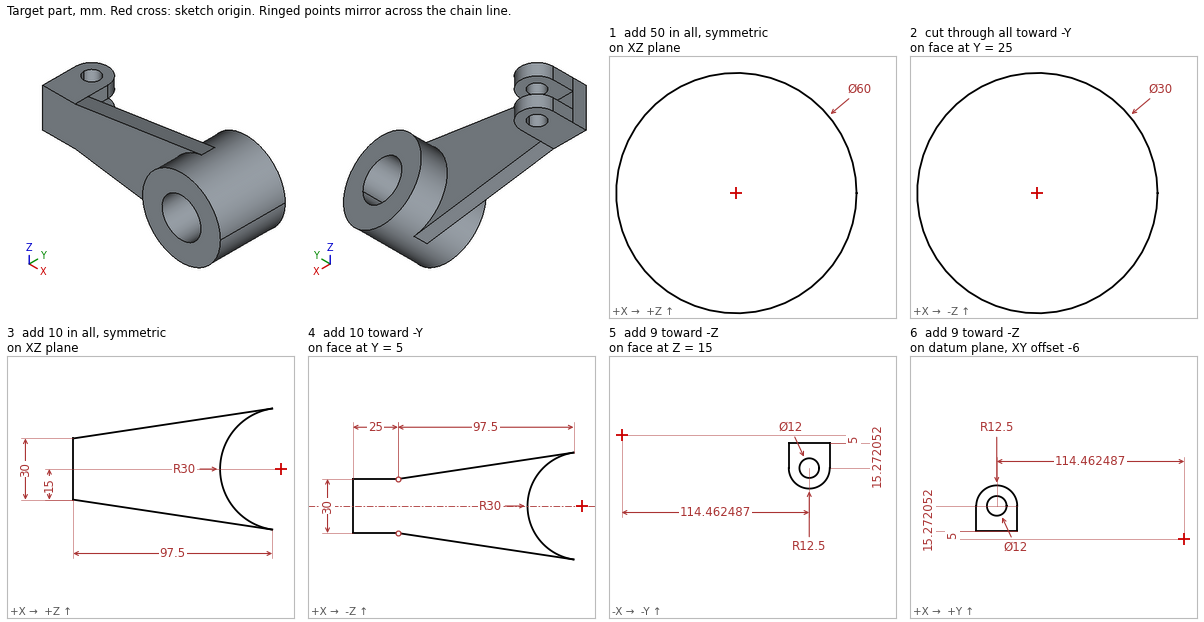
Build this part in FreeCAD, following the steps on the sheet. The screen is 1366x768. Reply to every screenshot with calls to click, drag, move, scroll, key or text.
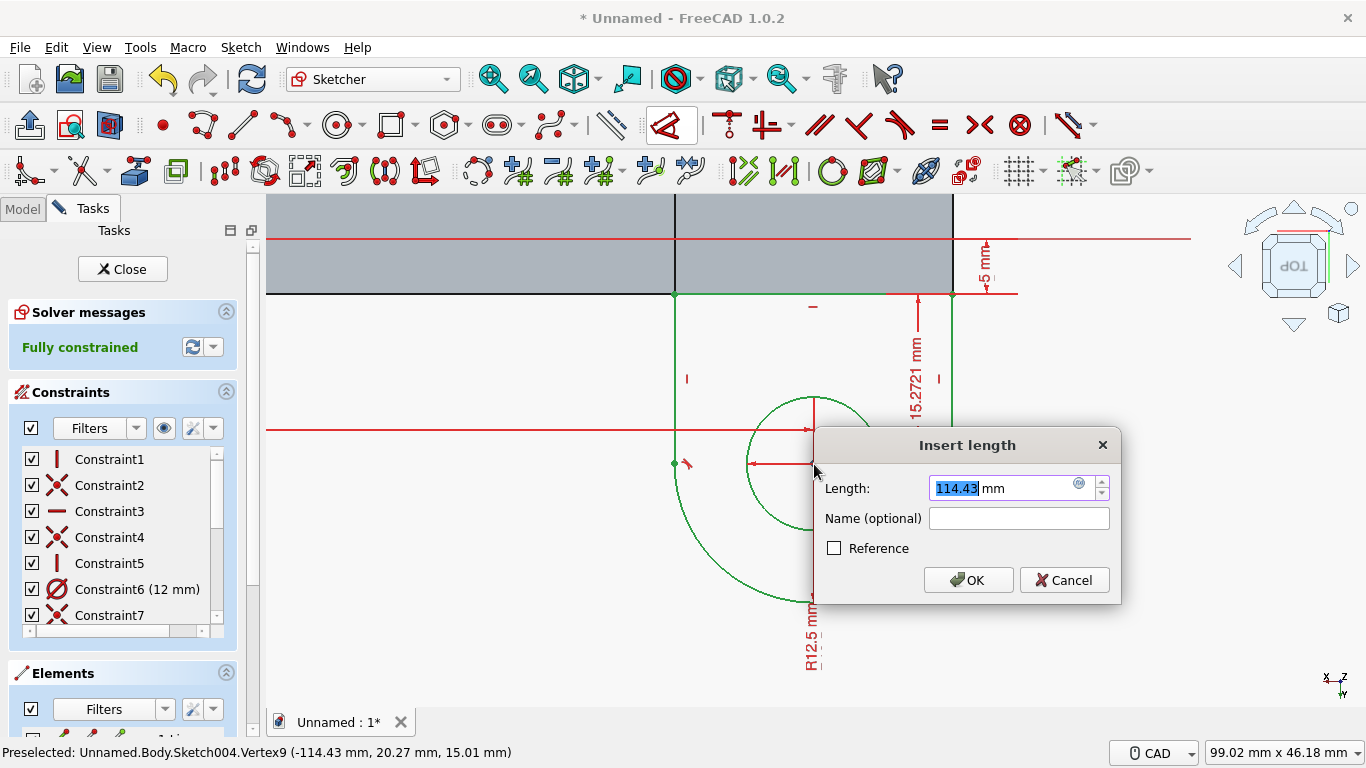
text(114.462487)
key(Return)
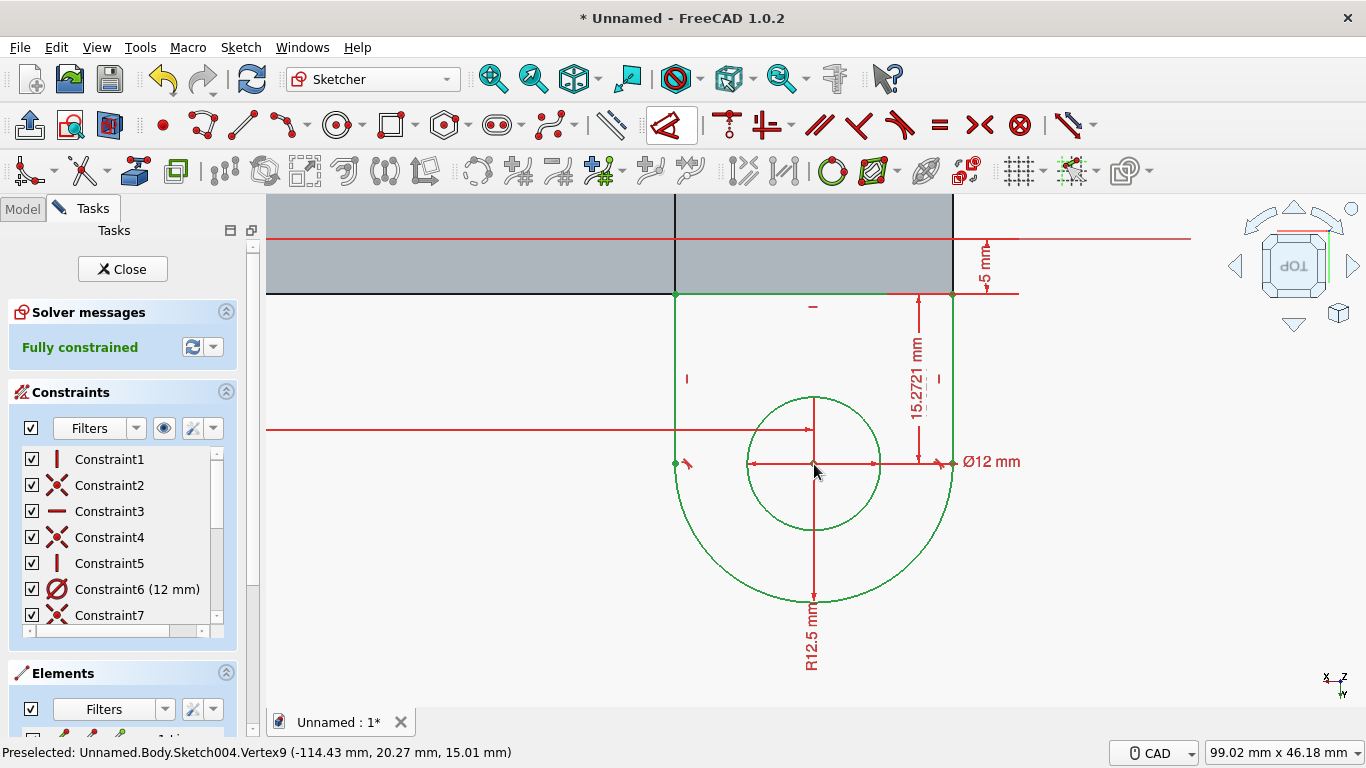
click(123, 269)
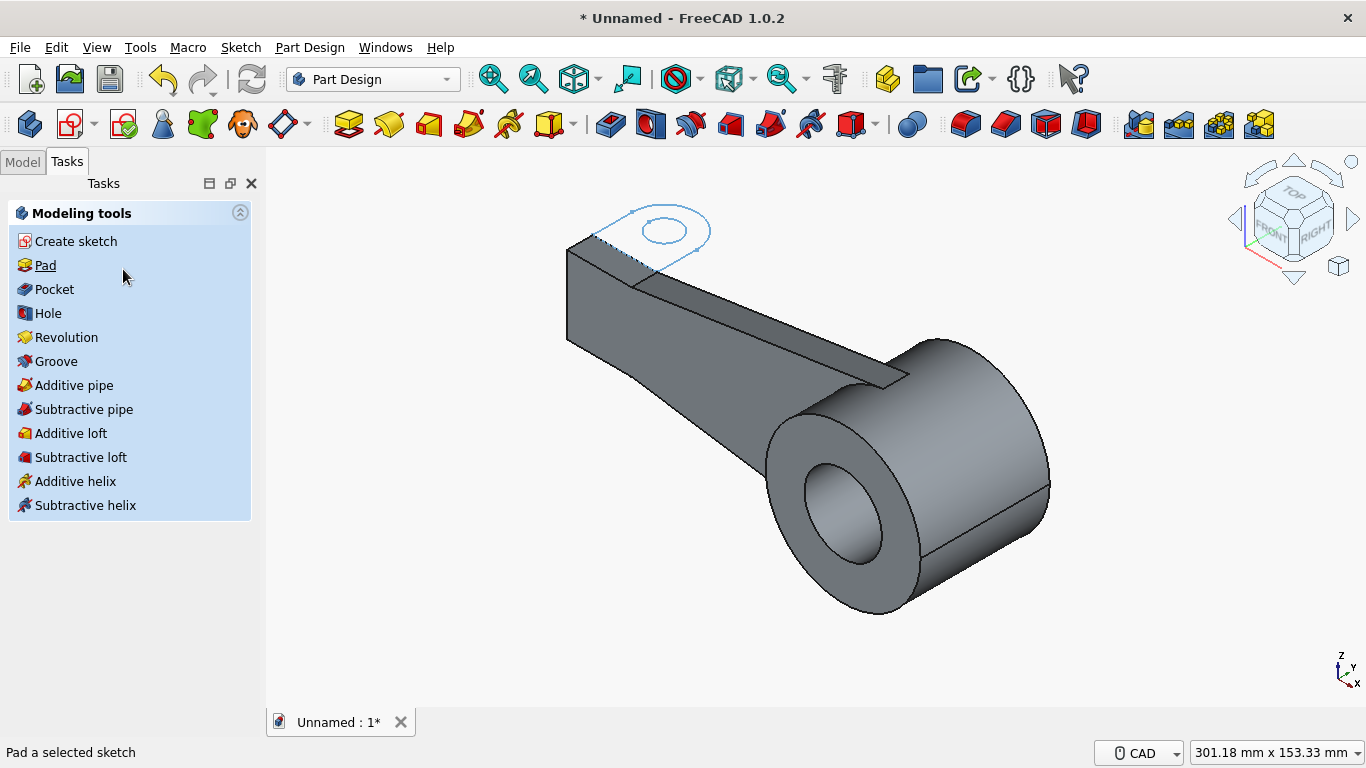
click(350, 124)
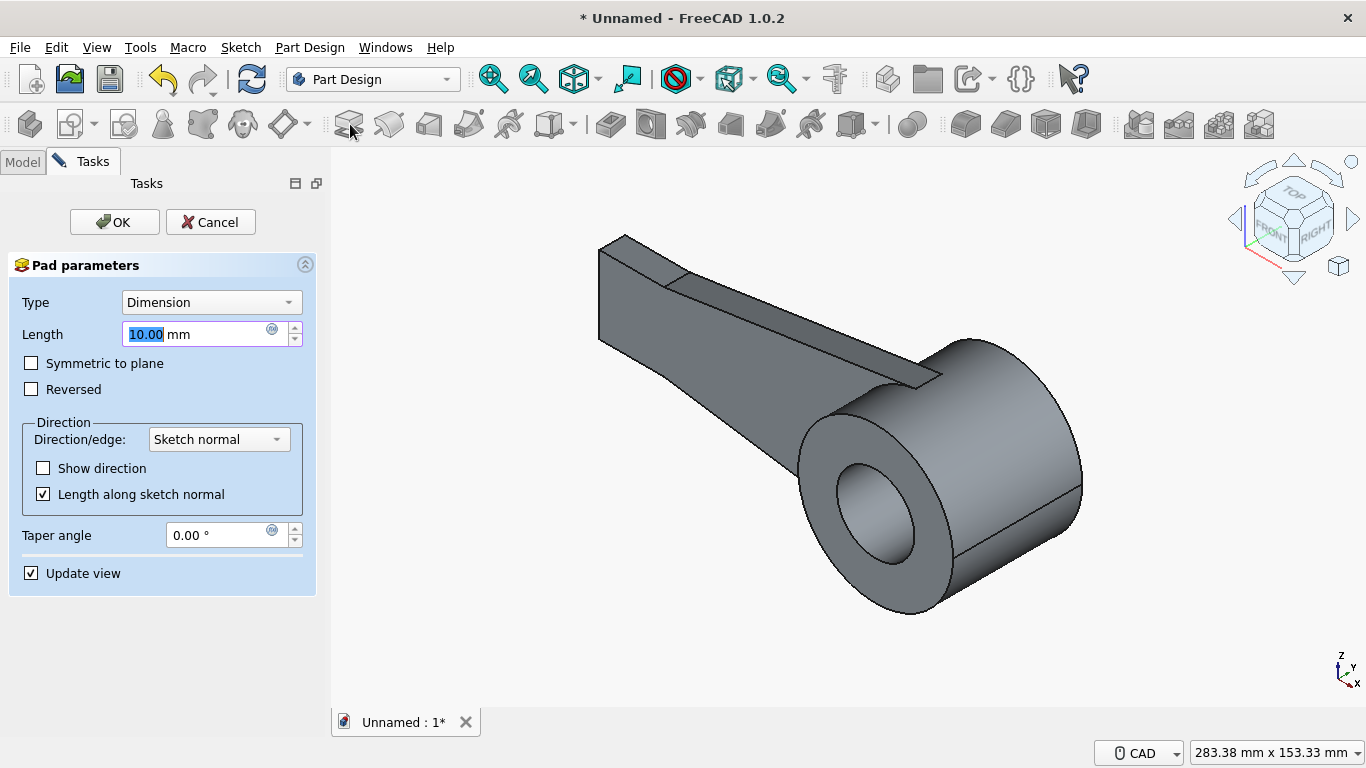
text(9)
key(Tab)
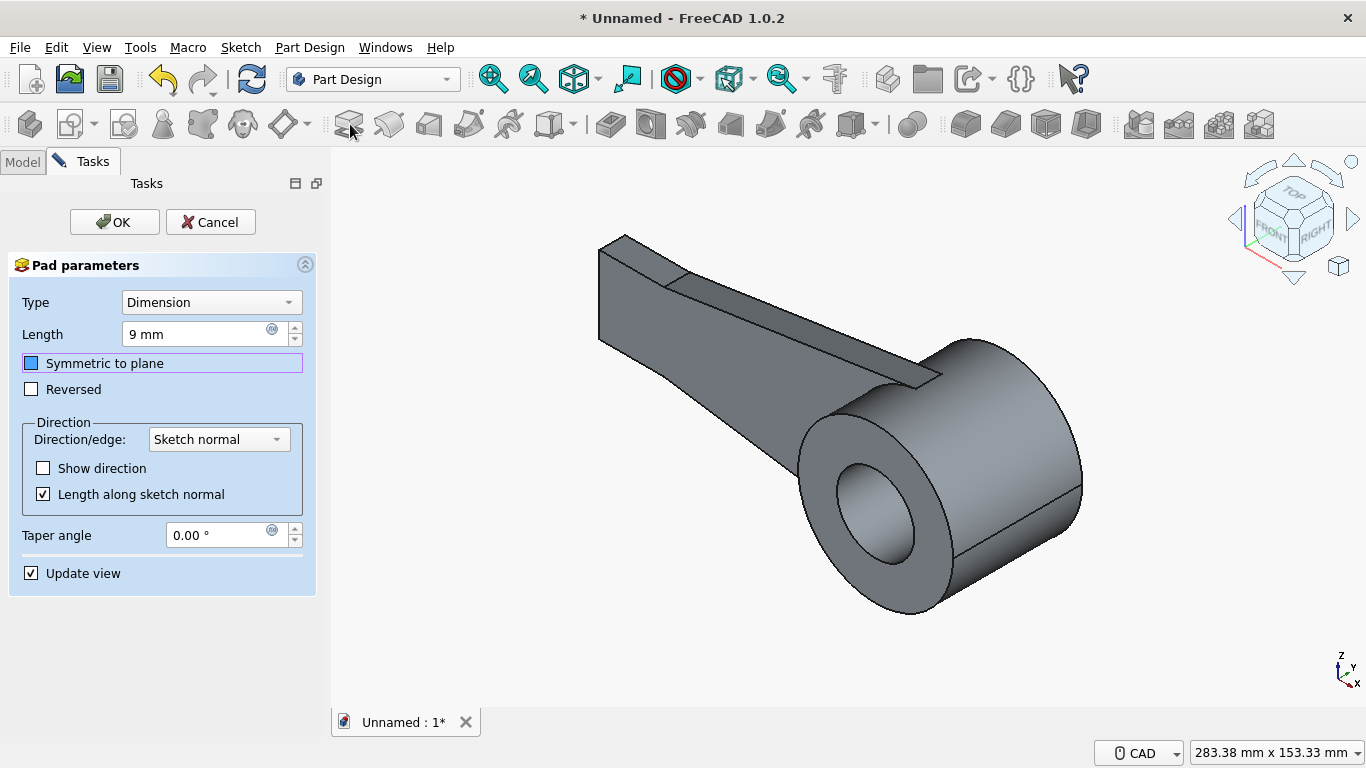
click(30, 389)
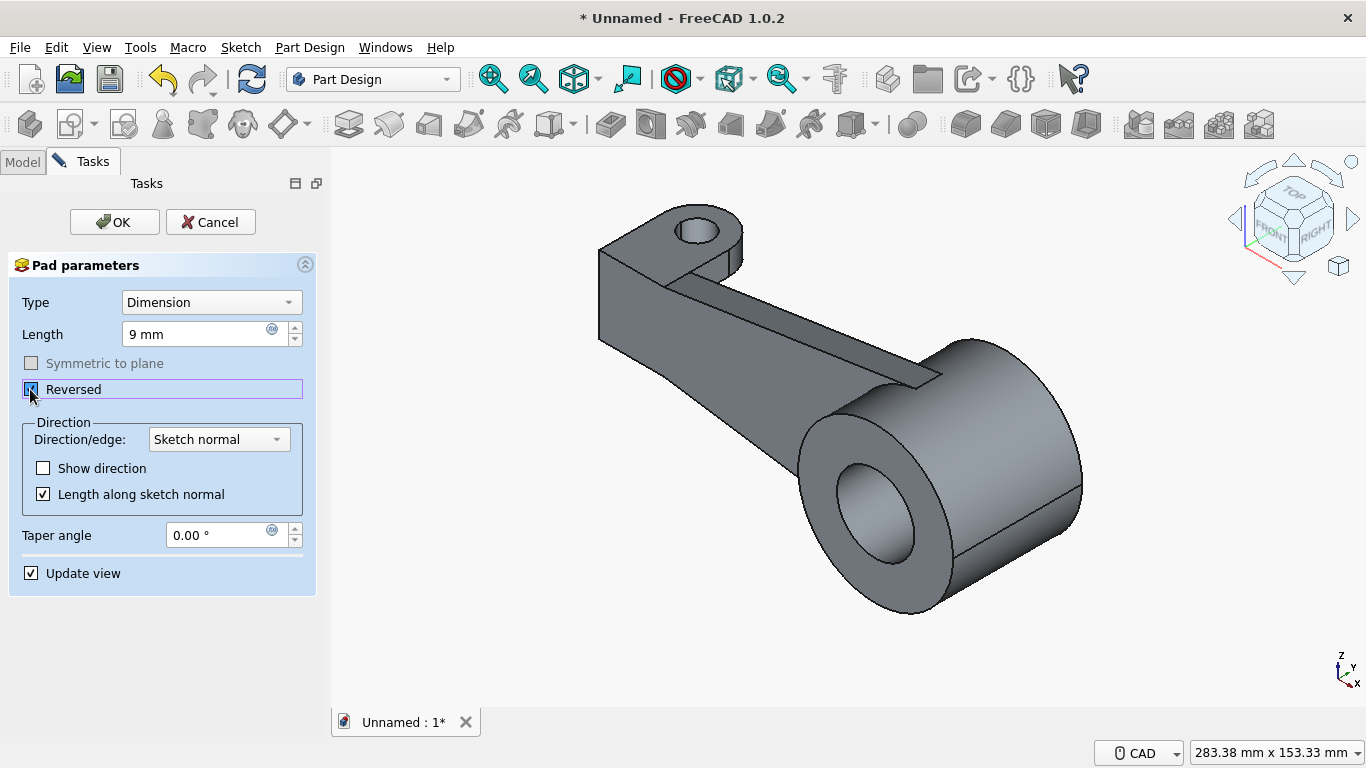
click(115, 222)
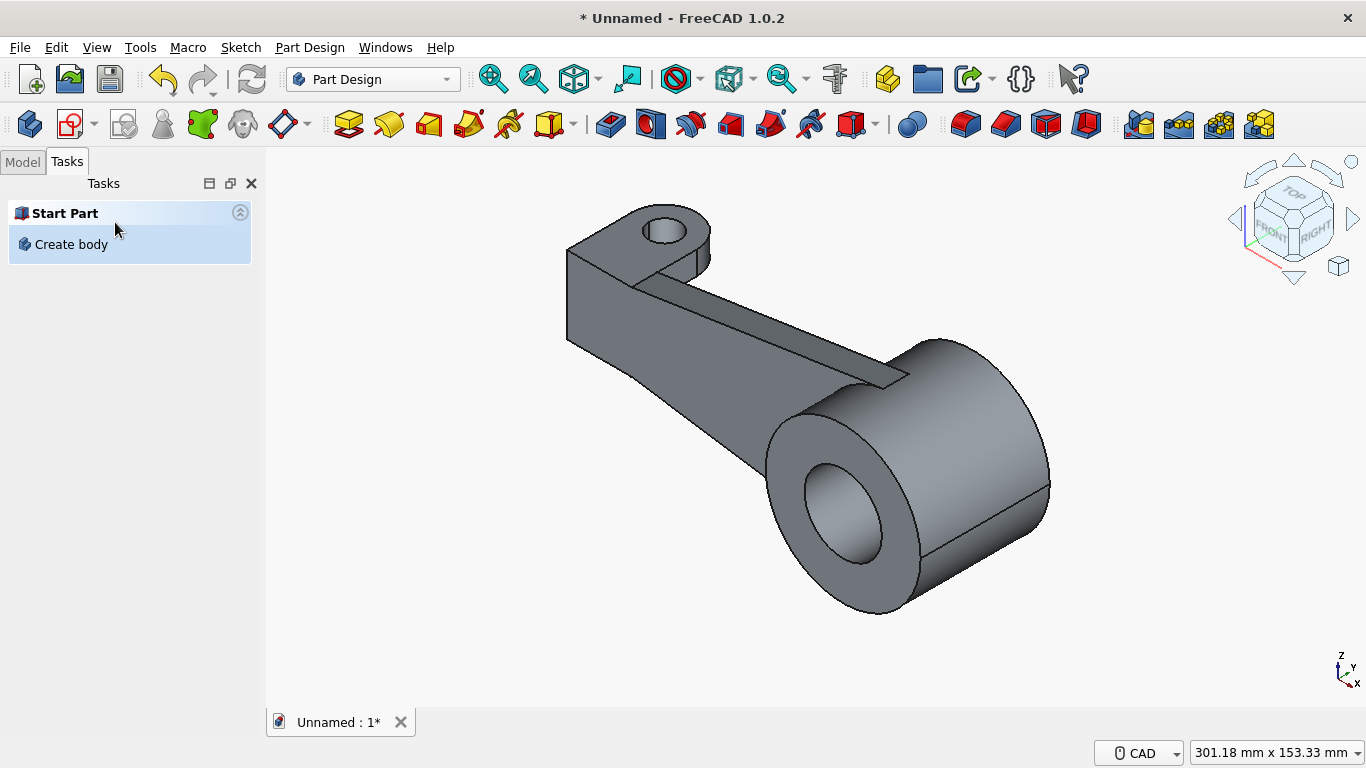
click(23, 161)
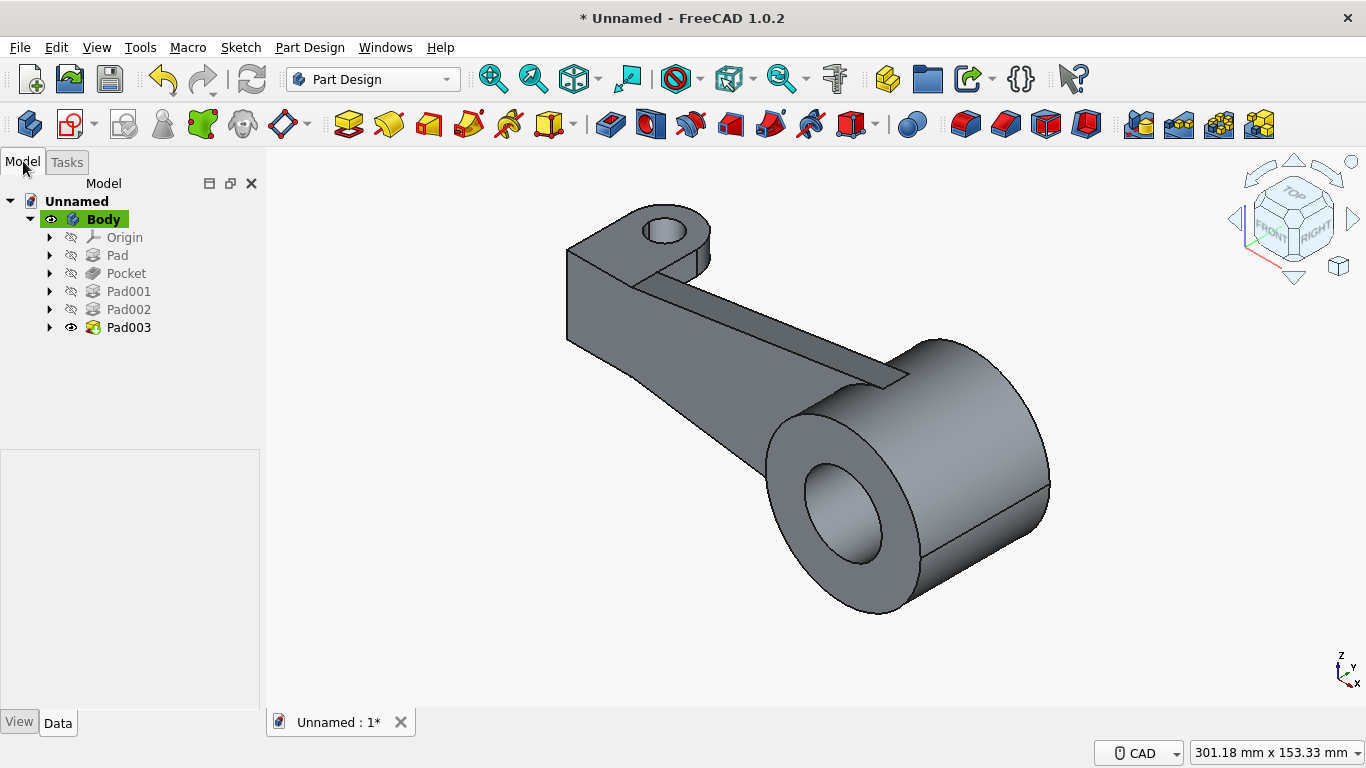
click(50, 237)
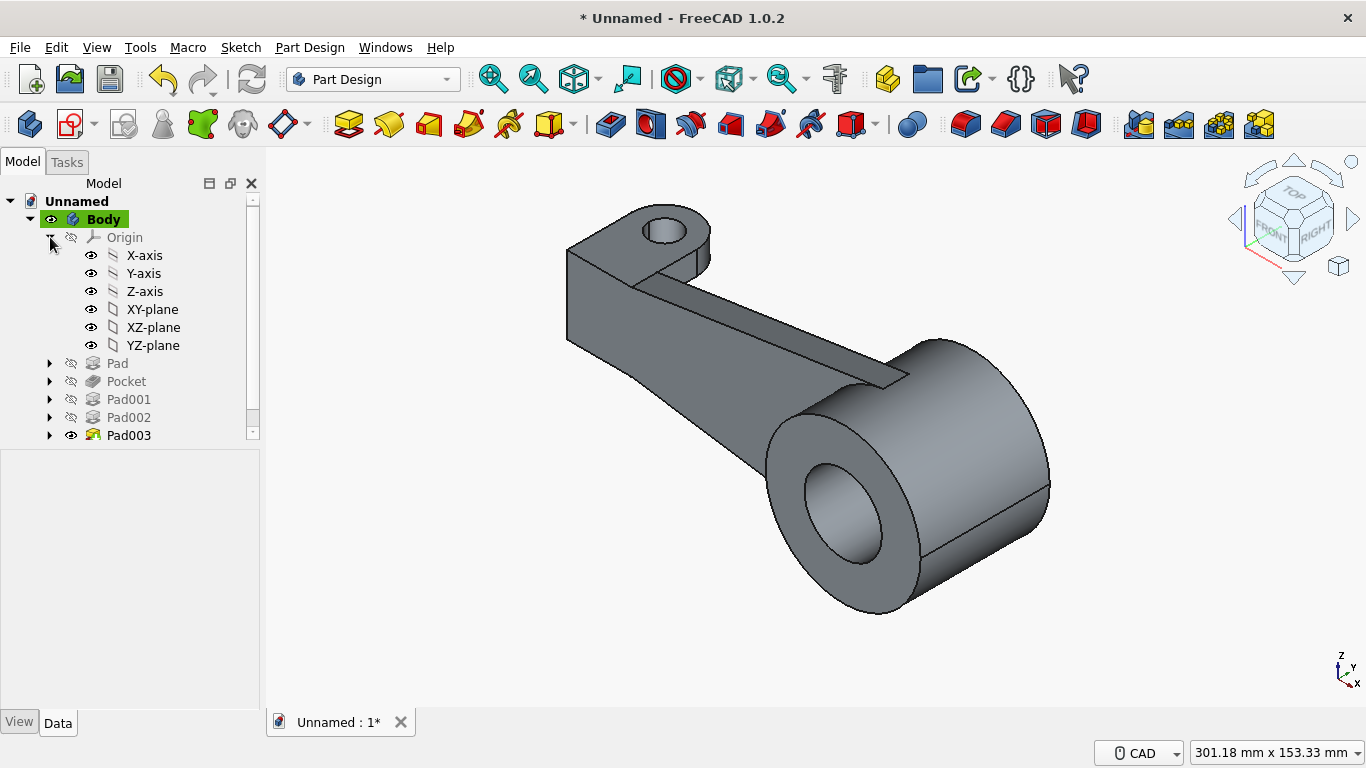
click(136, 309)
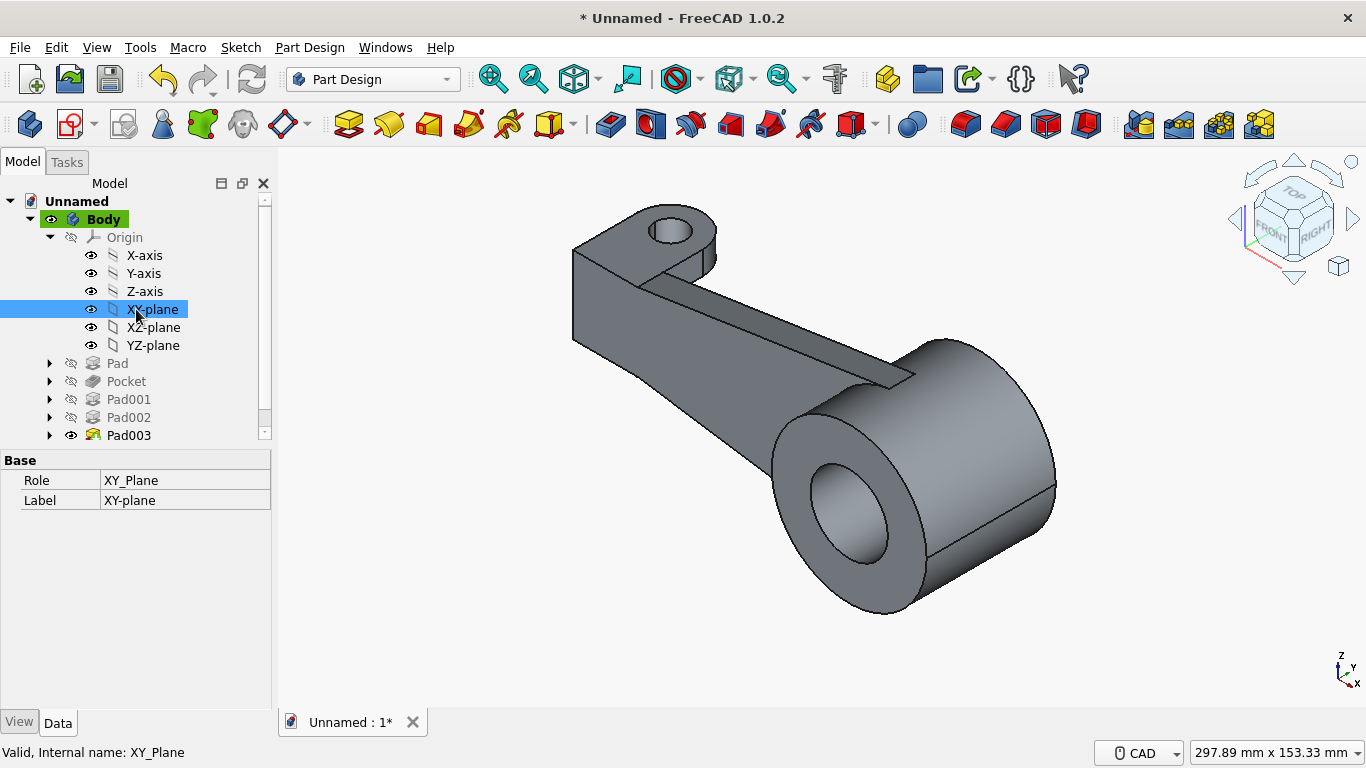
click(284, 124)